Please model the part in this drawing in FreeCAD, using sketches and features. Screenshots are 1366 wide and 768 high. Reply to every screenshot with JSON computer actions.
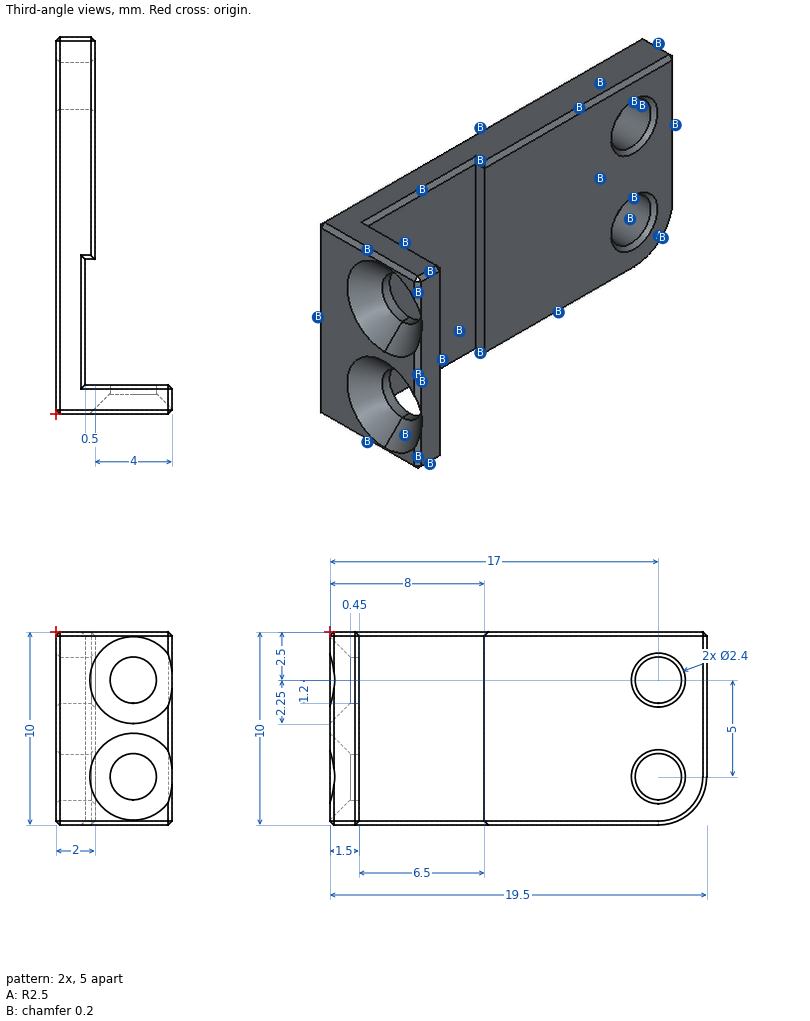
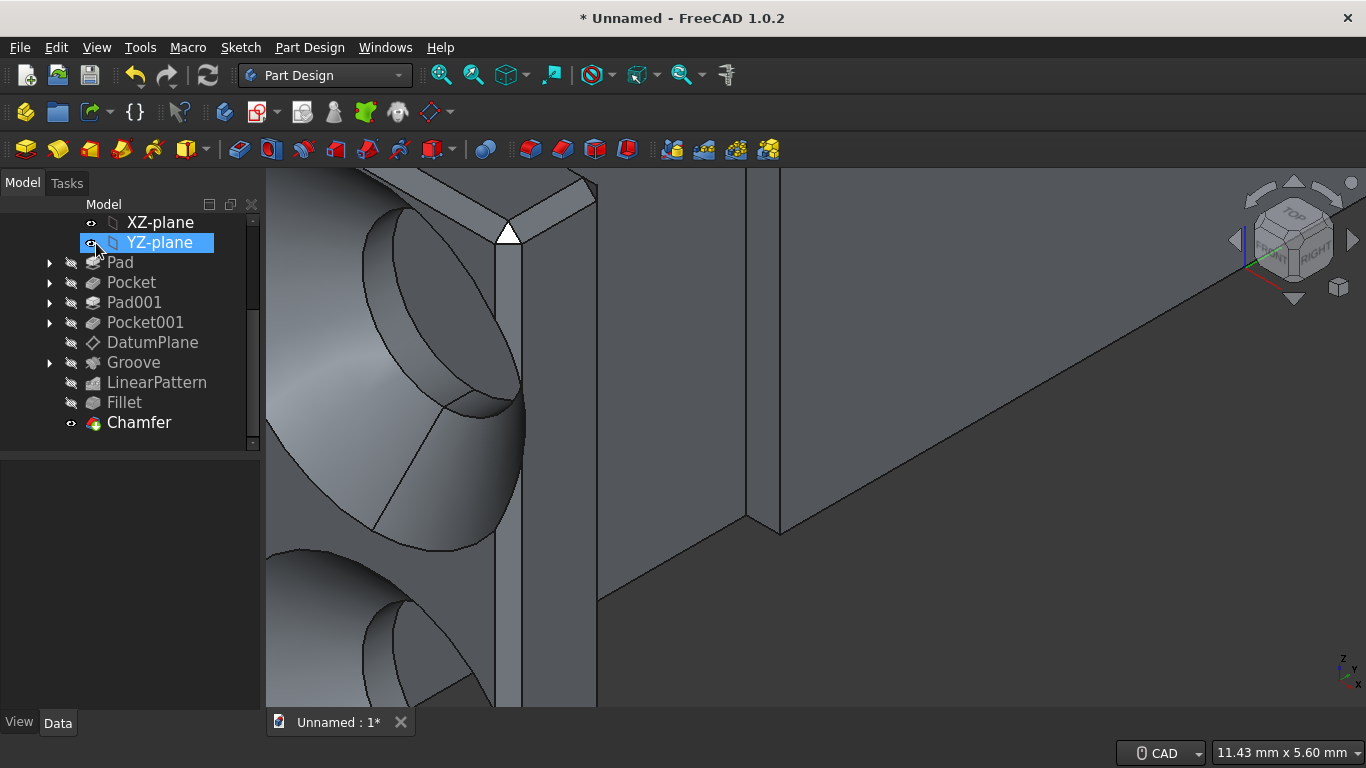
{"action": "left_click", "coordinate": [442, 76]}